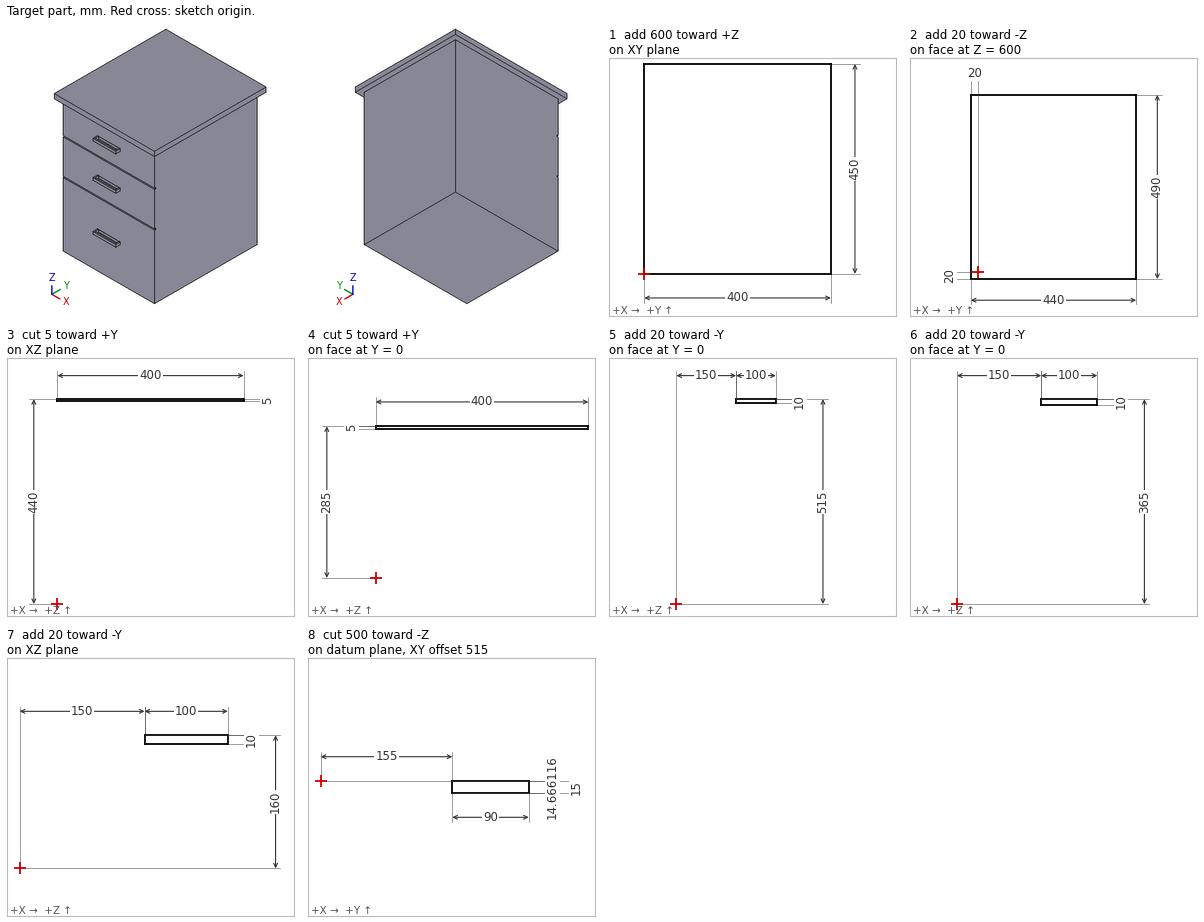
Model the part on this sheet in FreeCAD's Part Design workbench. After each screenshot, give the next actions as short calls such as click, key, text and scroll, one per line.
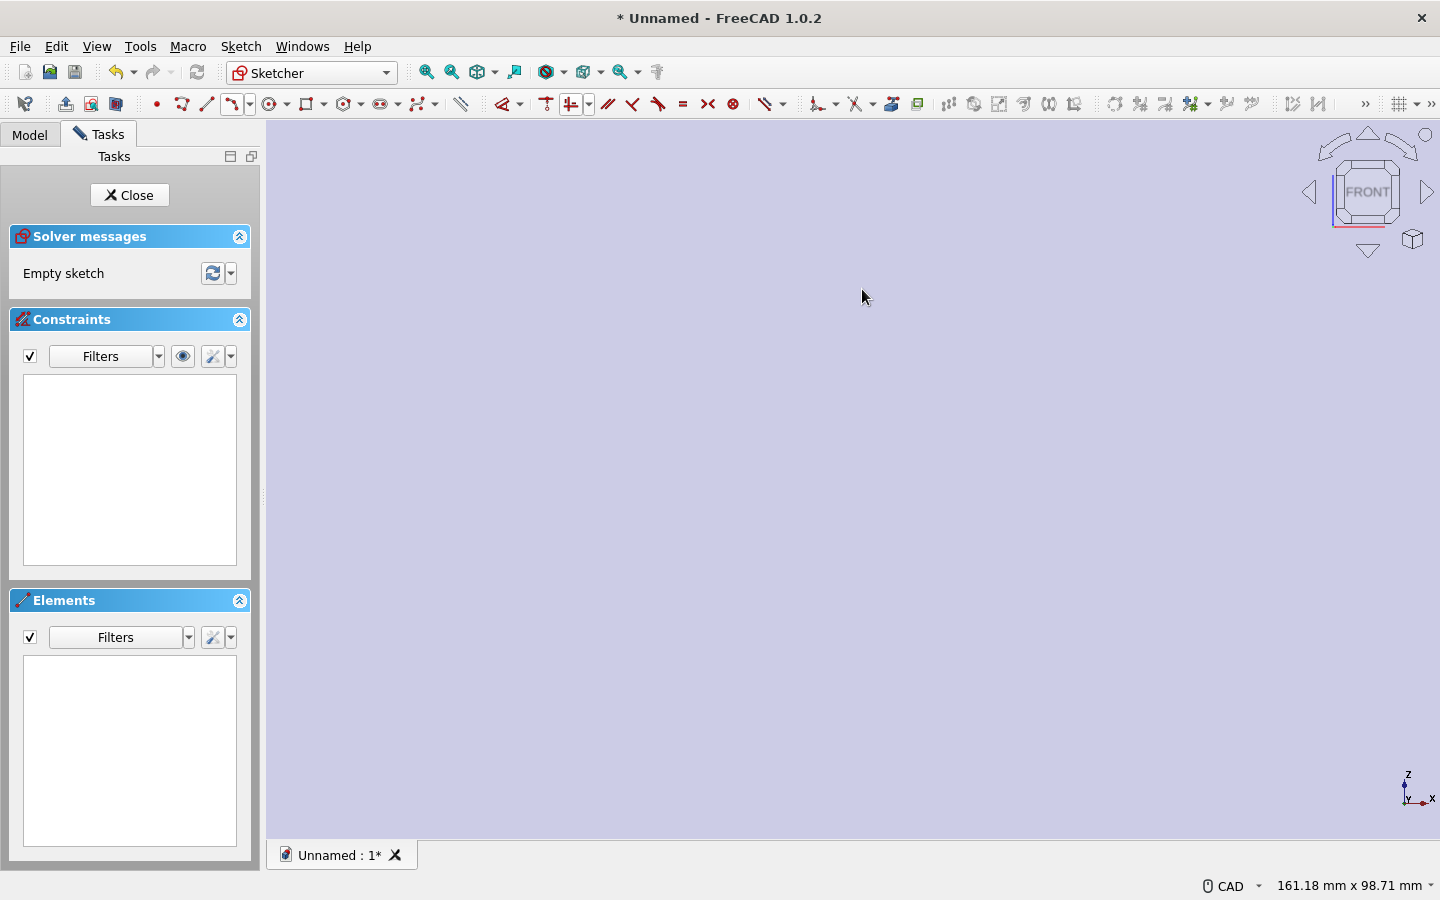
key(g)
key(r)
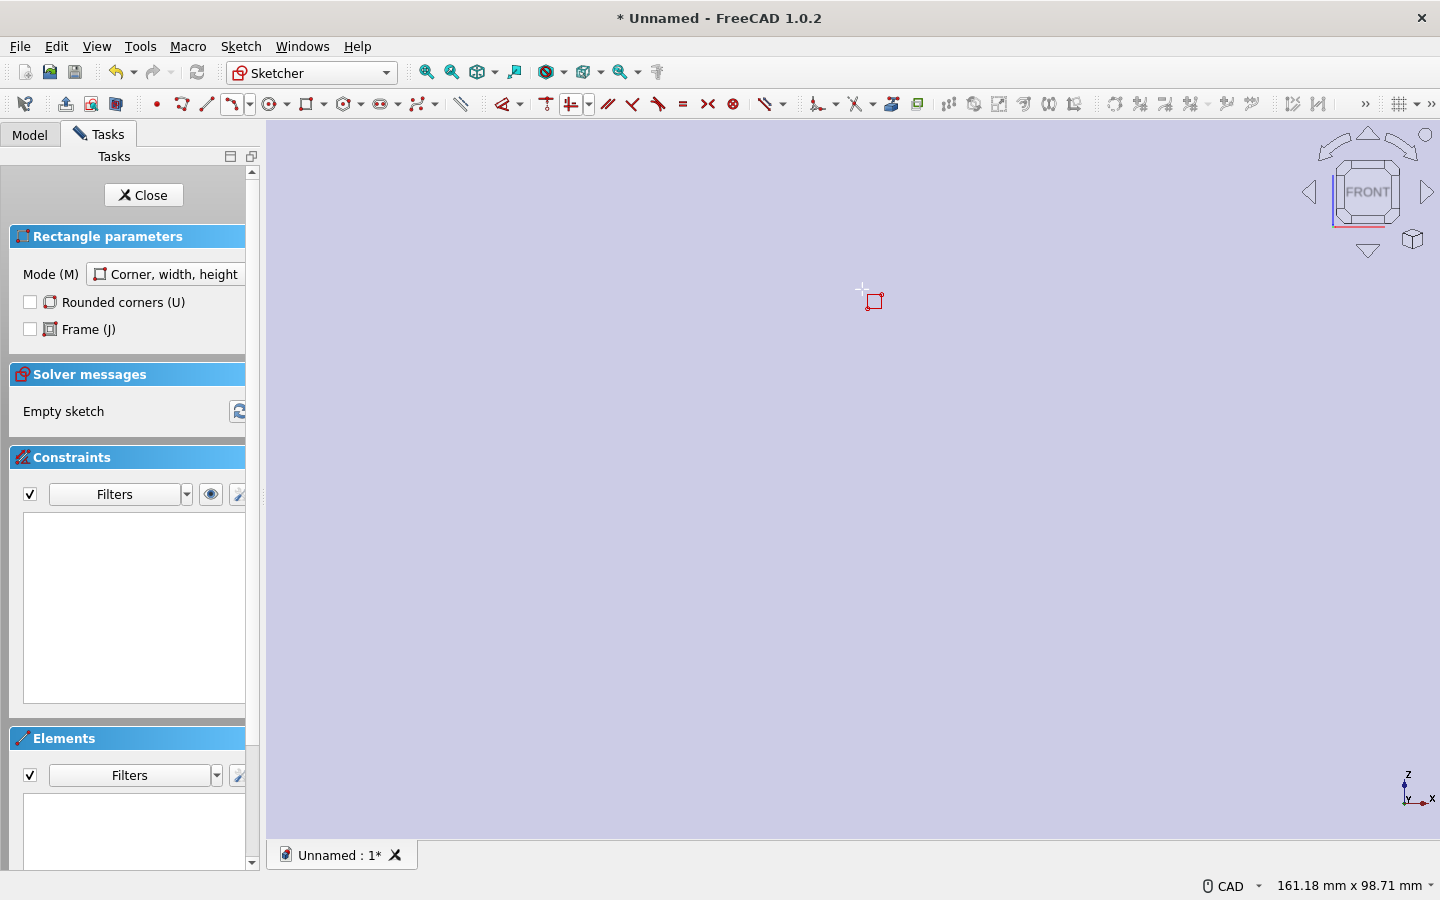
click(413, 440)
move(1141, 513)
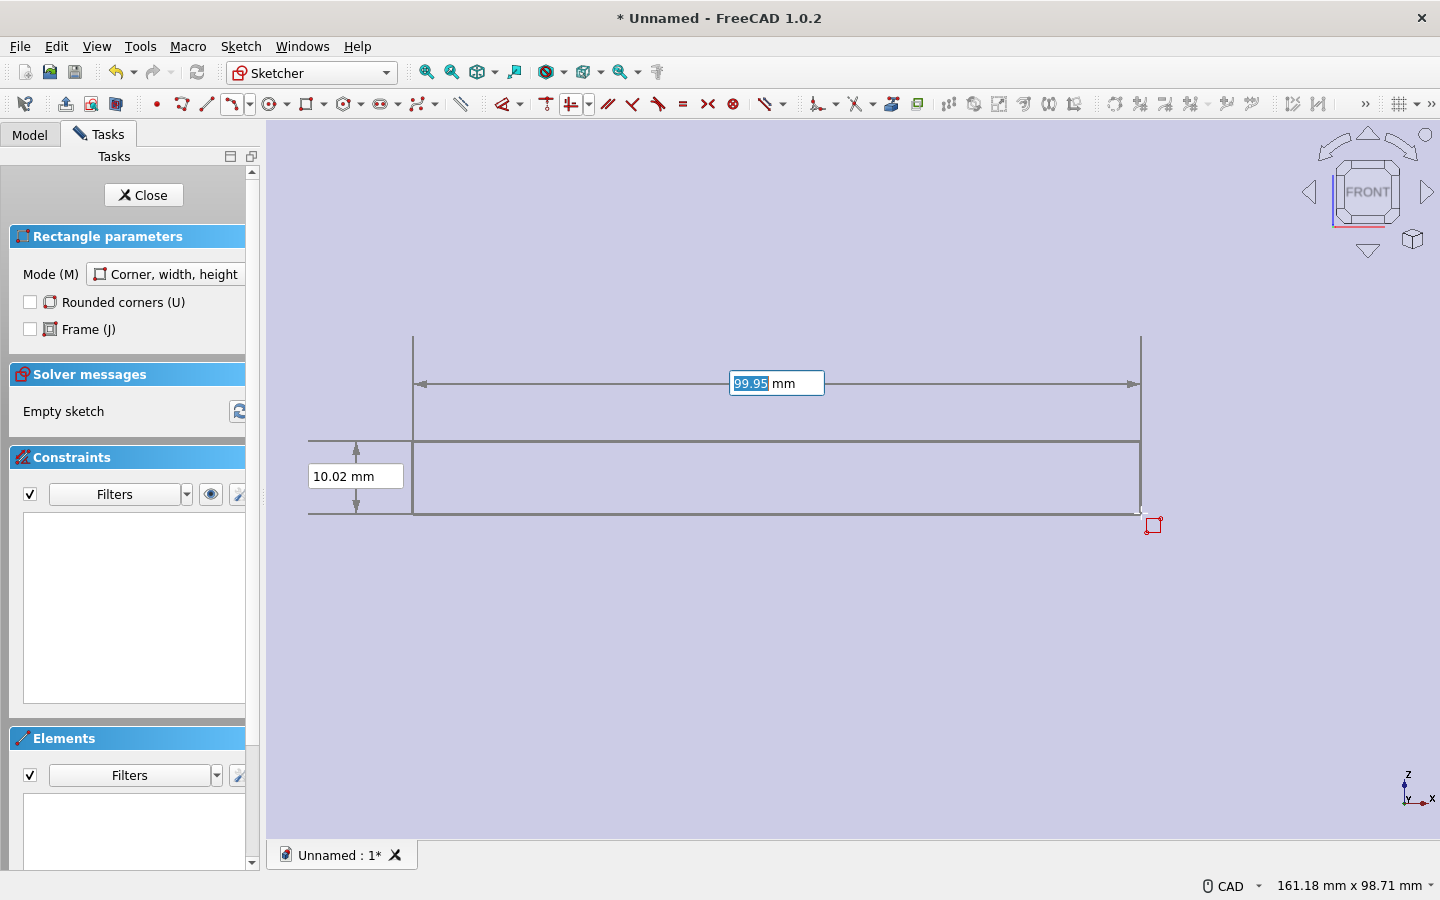
text(100)
key(Tab)
text(10)
key(Return)
key(Escape)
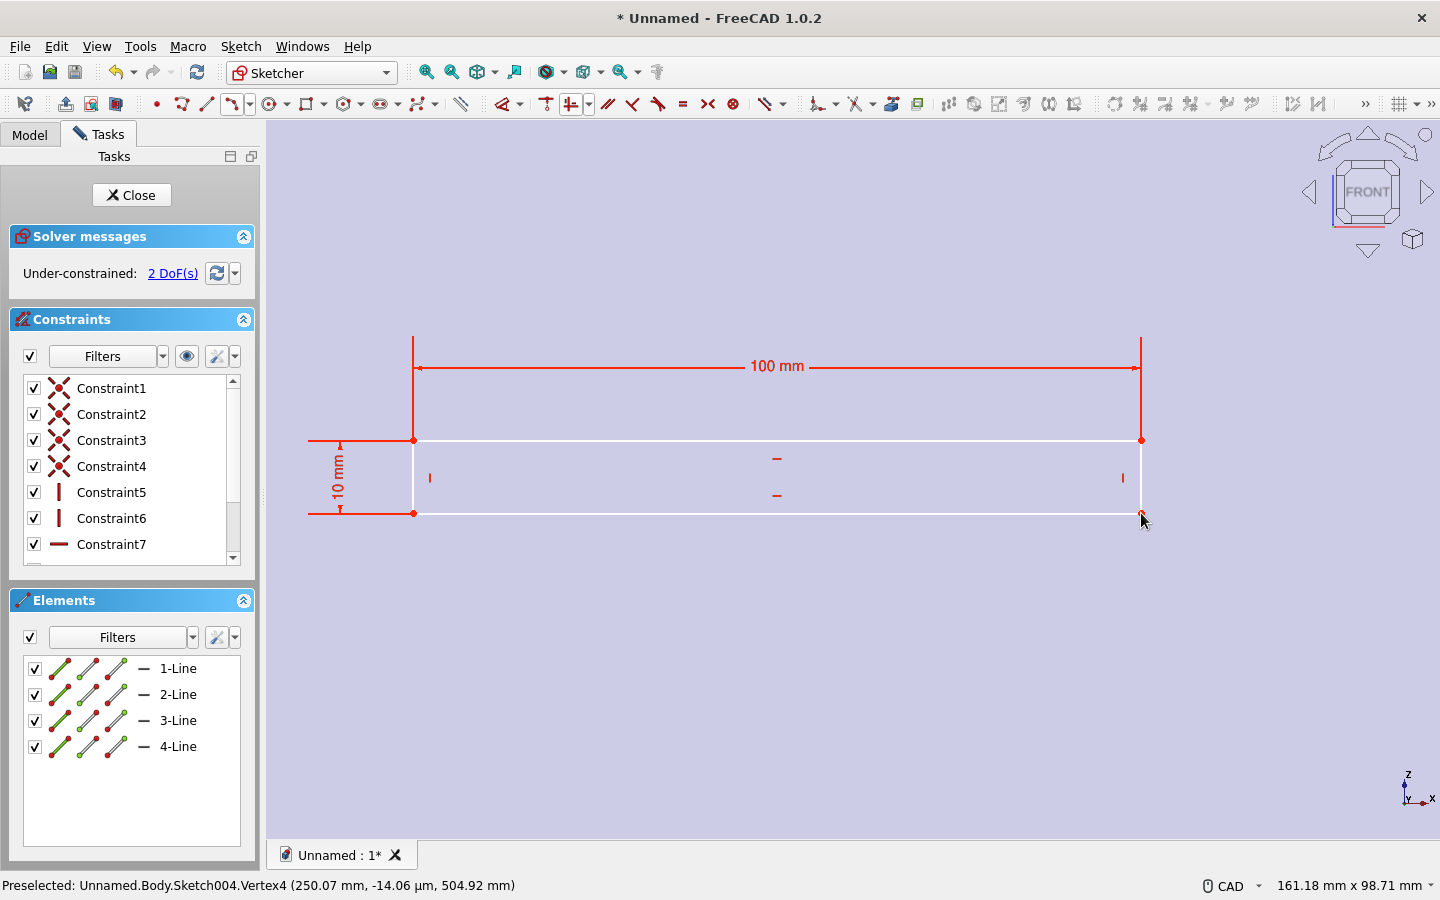
click(502, 104)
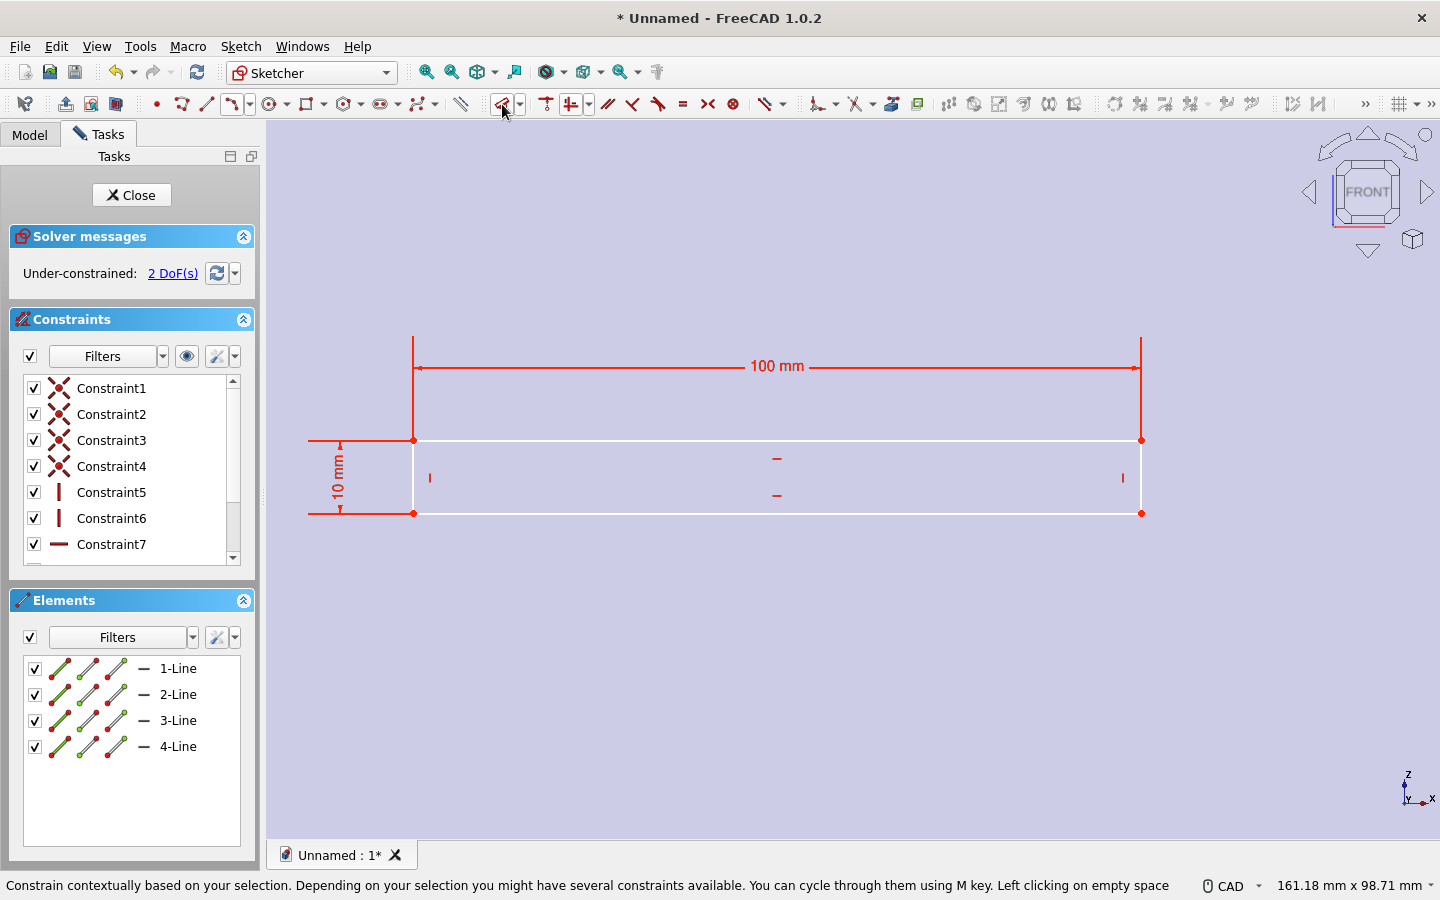
click(413, 441)
click(354, 407)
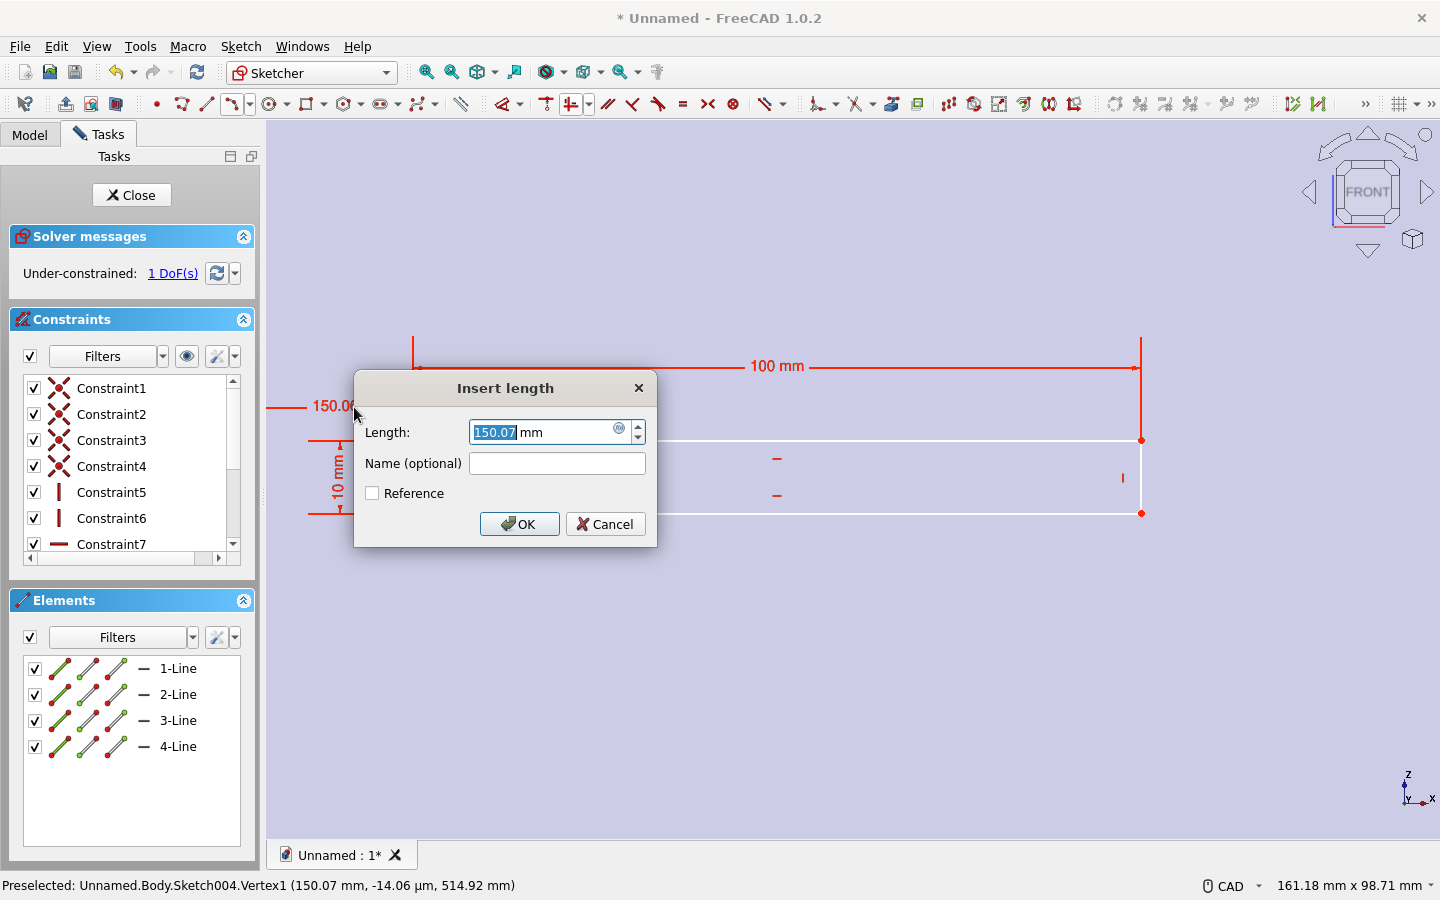
text(150)
key(Return)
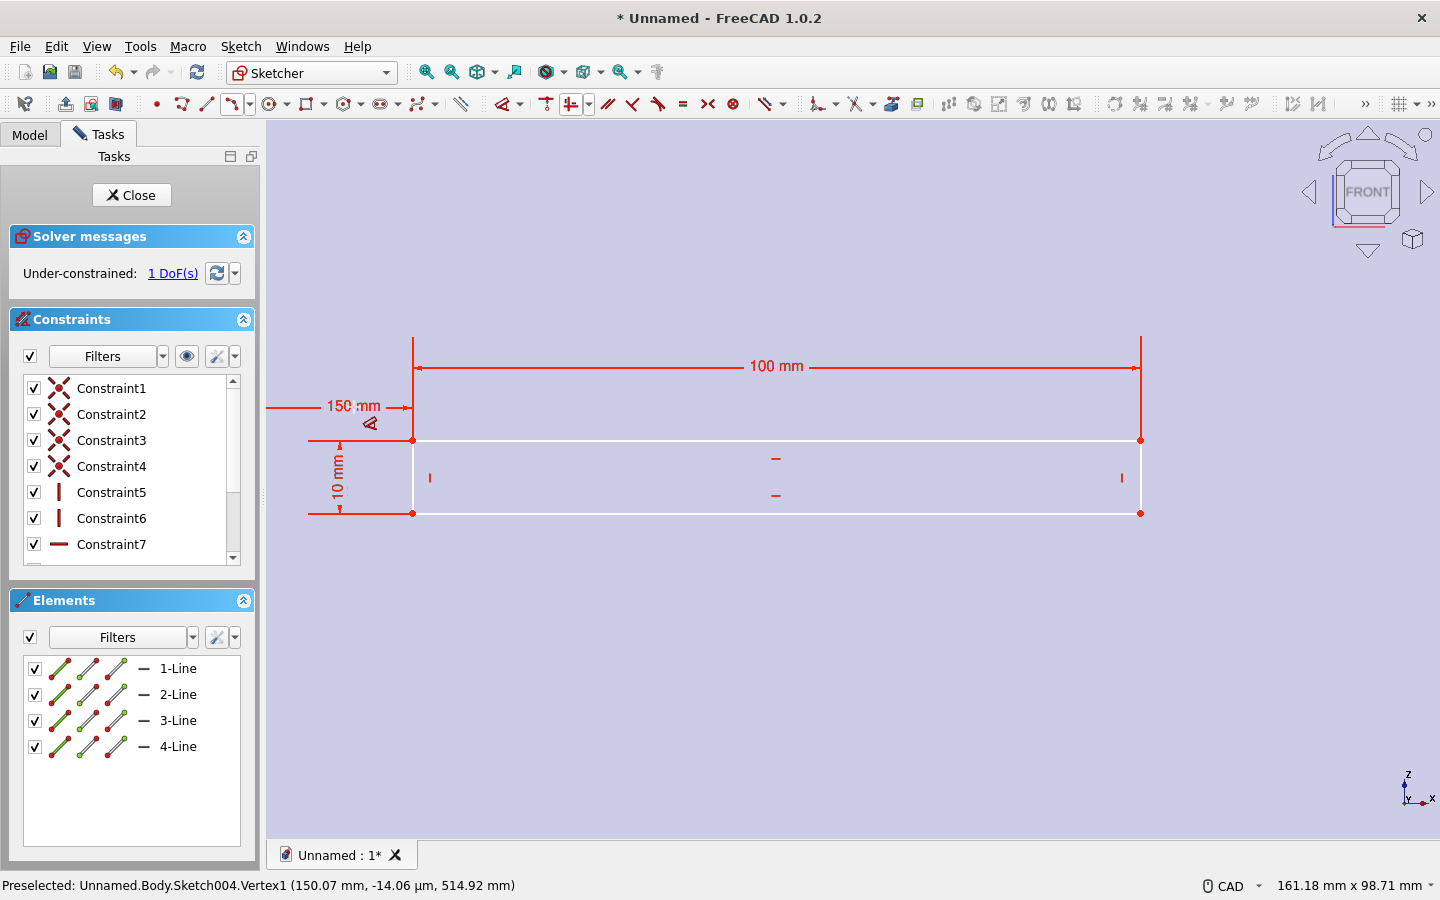
click(413, 441)
click(447, 626)